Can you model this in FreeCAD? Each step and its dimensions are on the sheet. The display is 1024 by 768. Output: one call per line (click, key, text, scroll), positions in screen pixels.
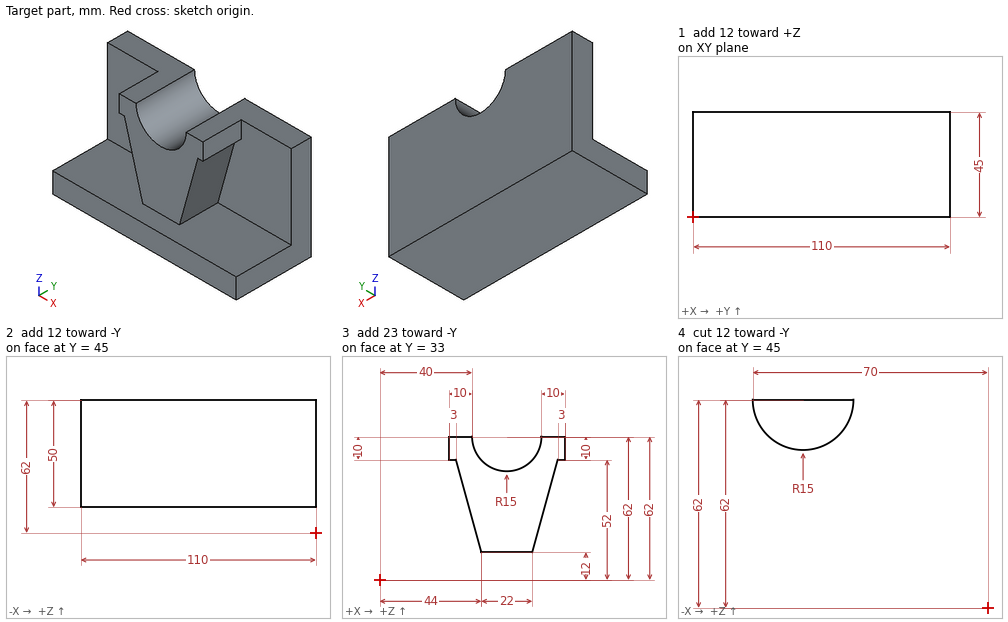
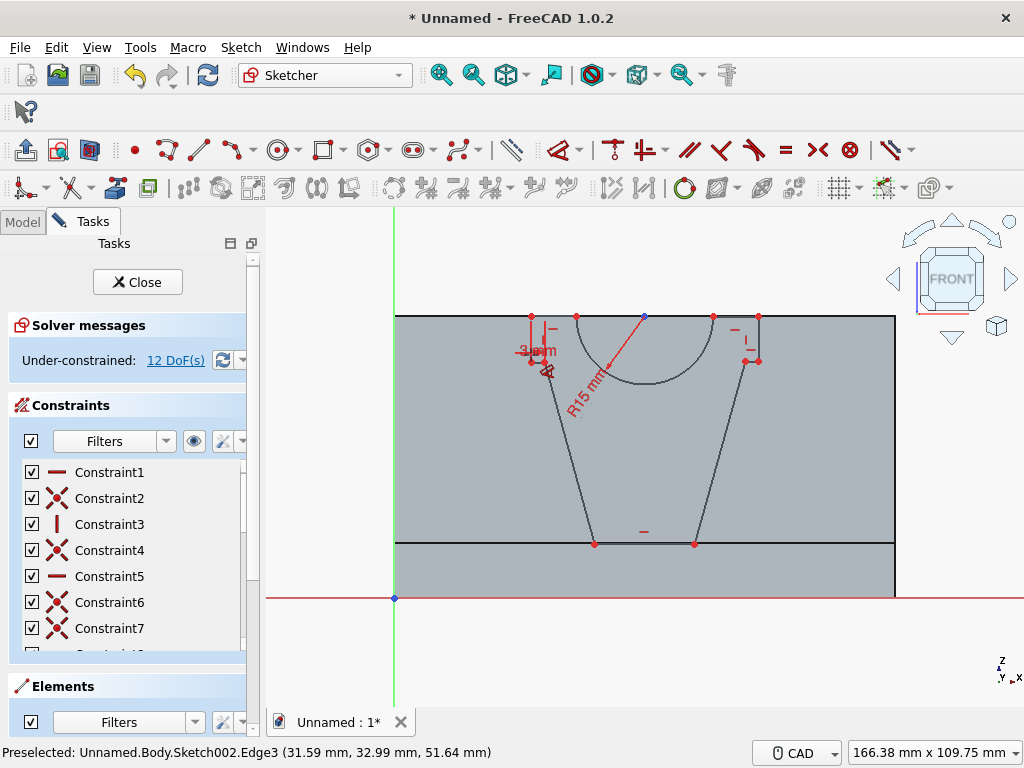
scroll(749, 362, up, 7)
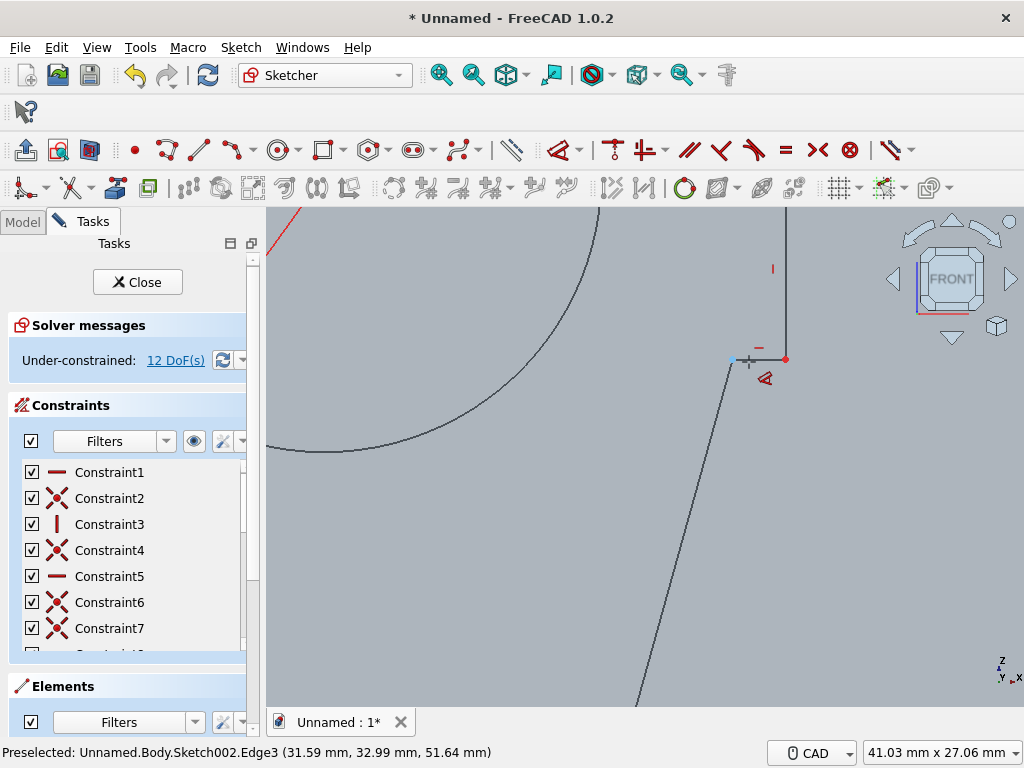
click(748, 360)
click(759, 326)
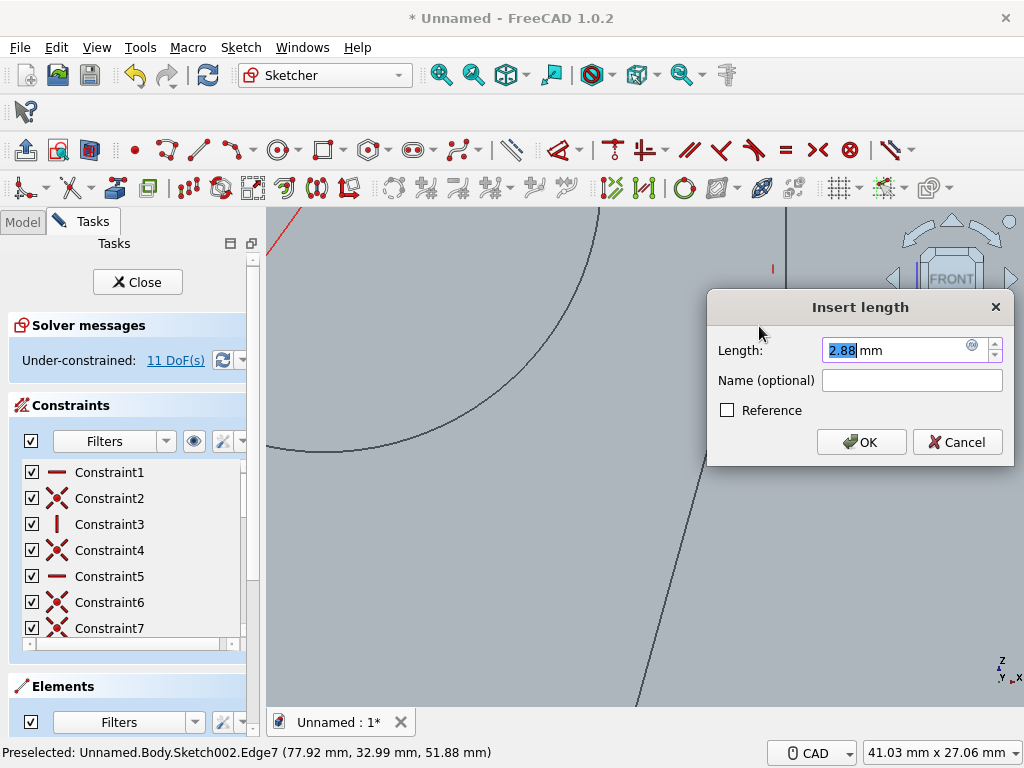
text(3)
key(Return)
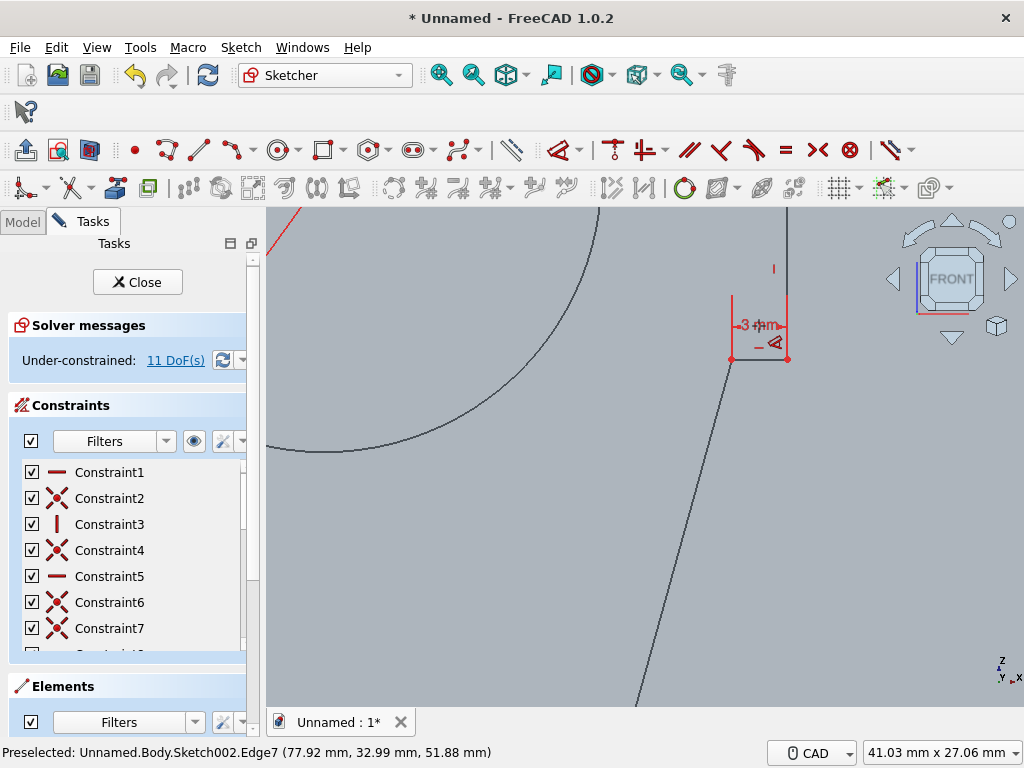
scroll(750, 362, down, 7)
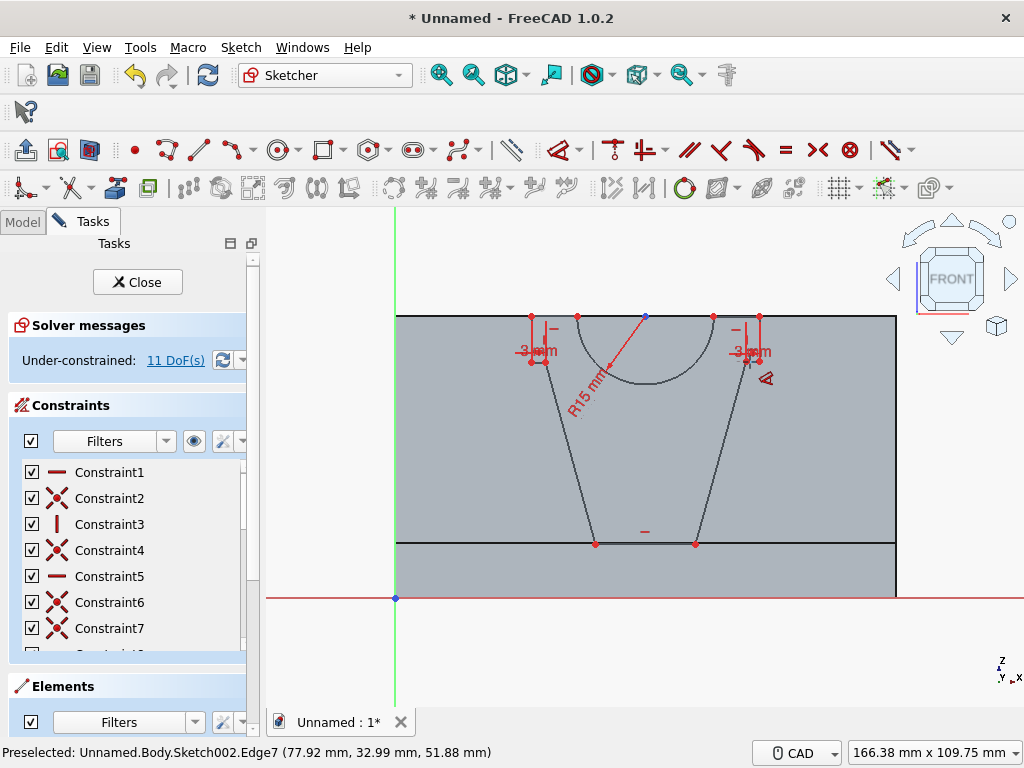
click(564, 316)
click(555, 282)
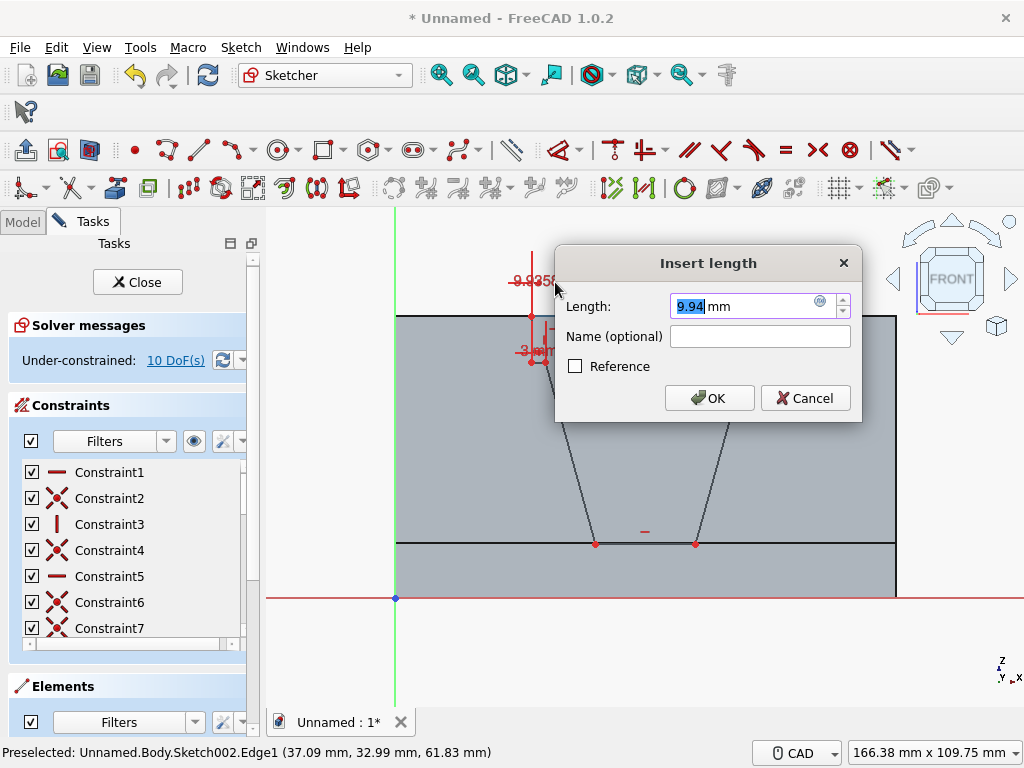
text(10)
key(Return)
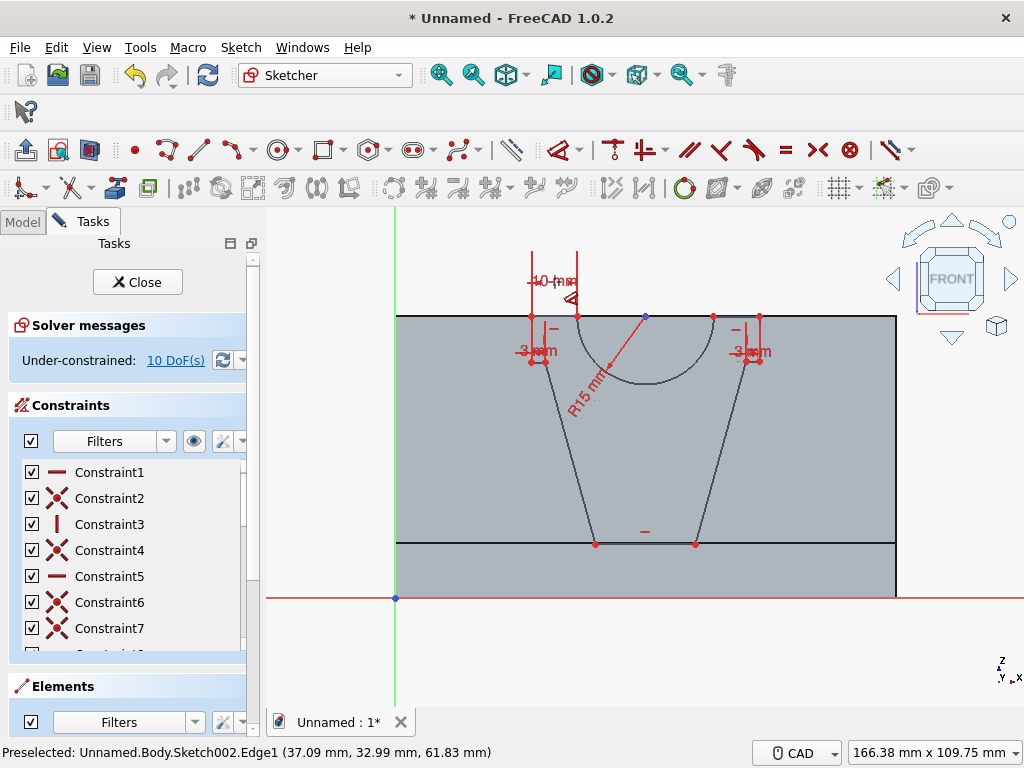
click(532, 330)
click(498, 329)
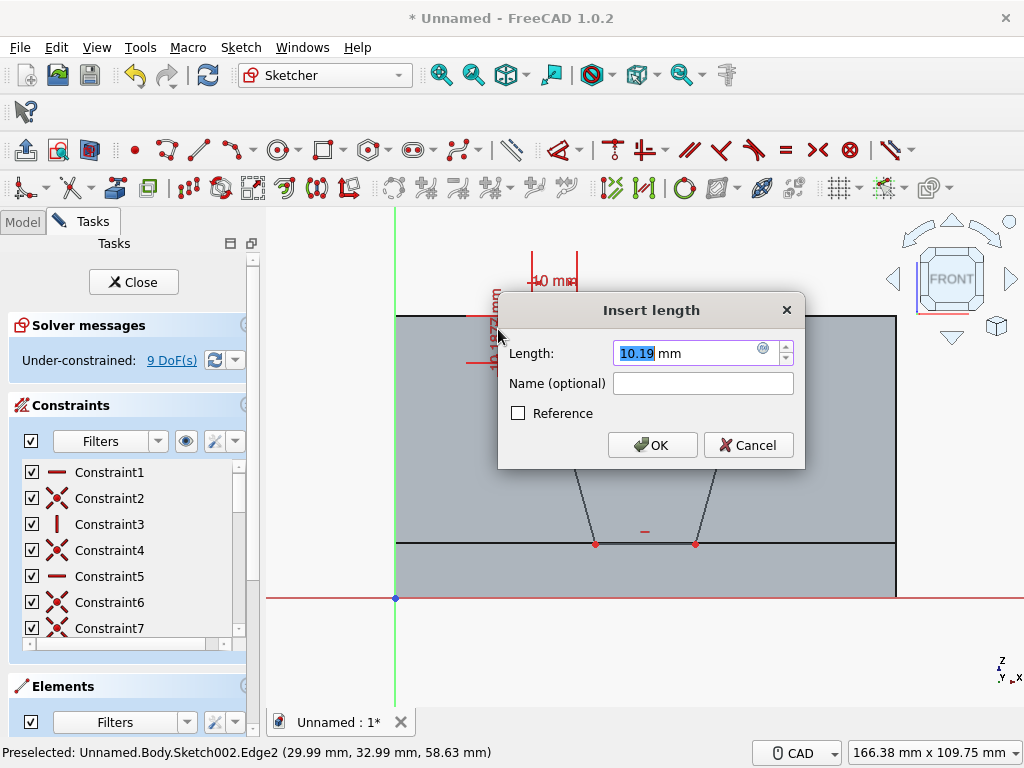
text(10)
key(Return)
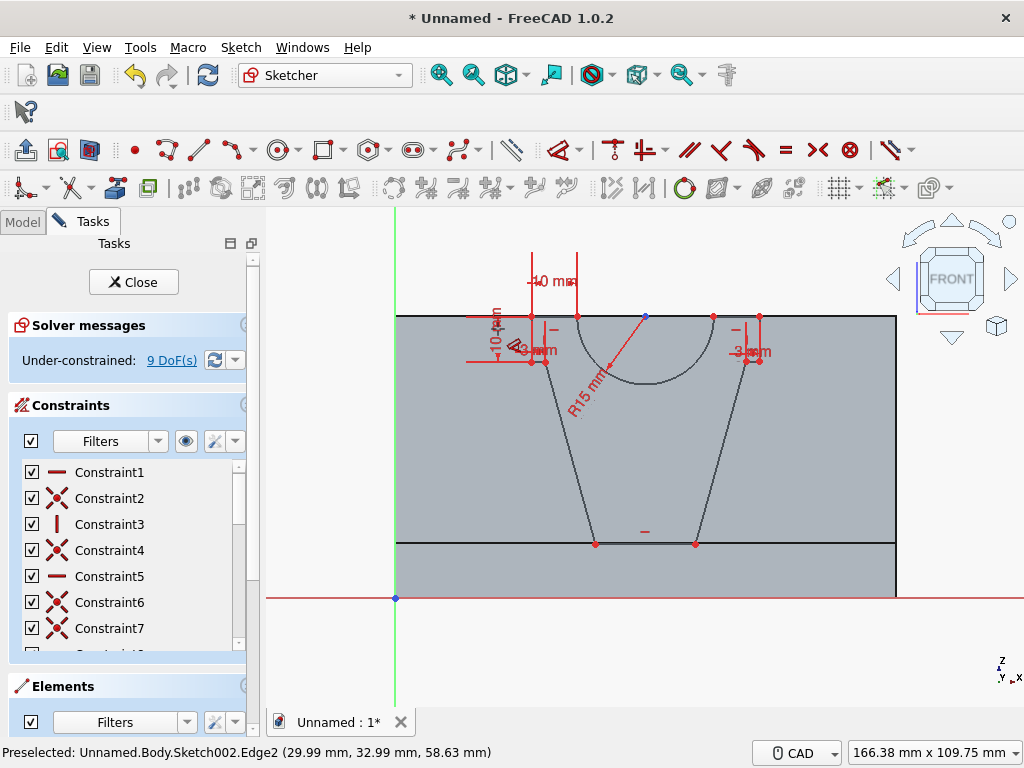
click(625, 544)
click(645, 578)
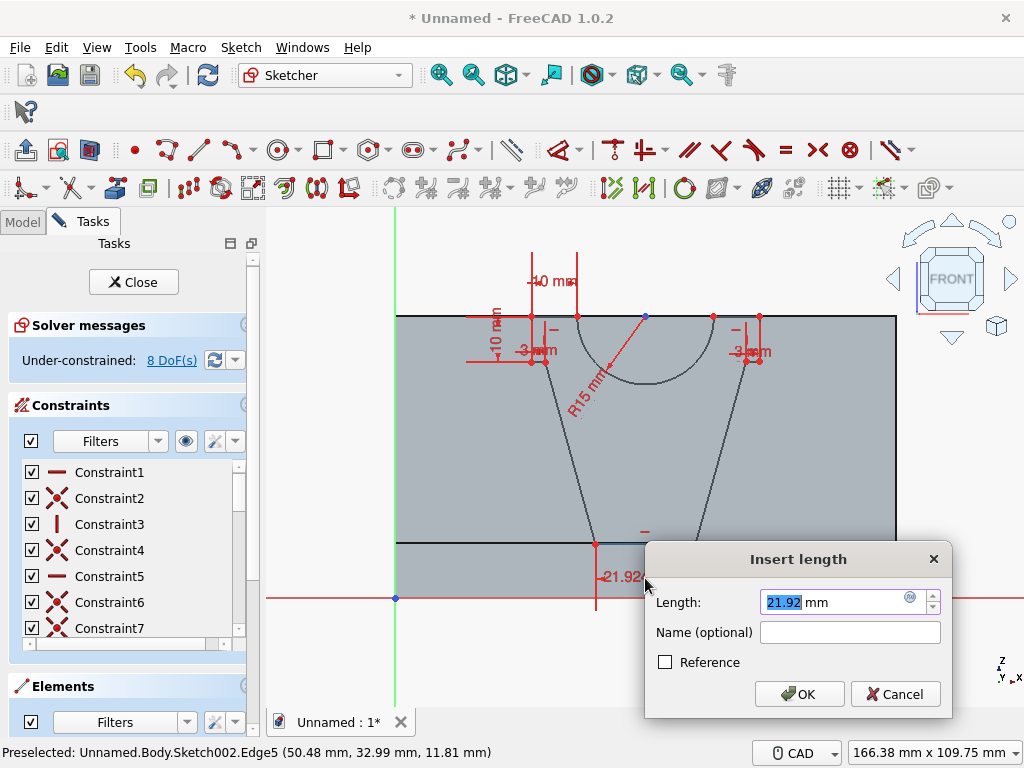
text(22)
key(Return)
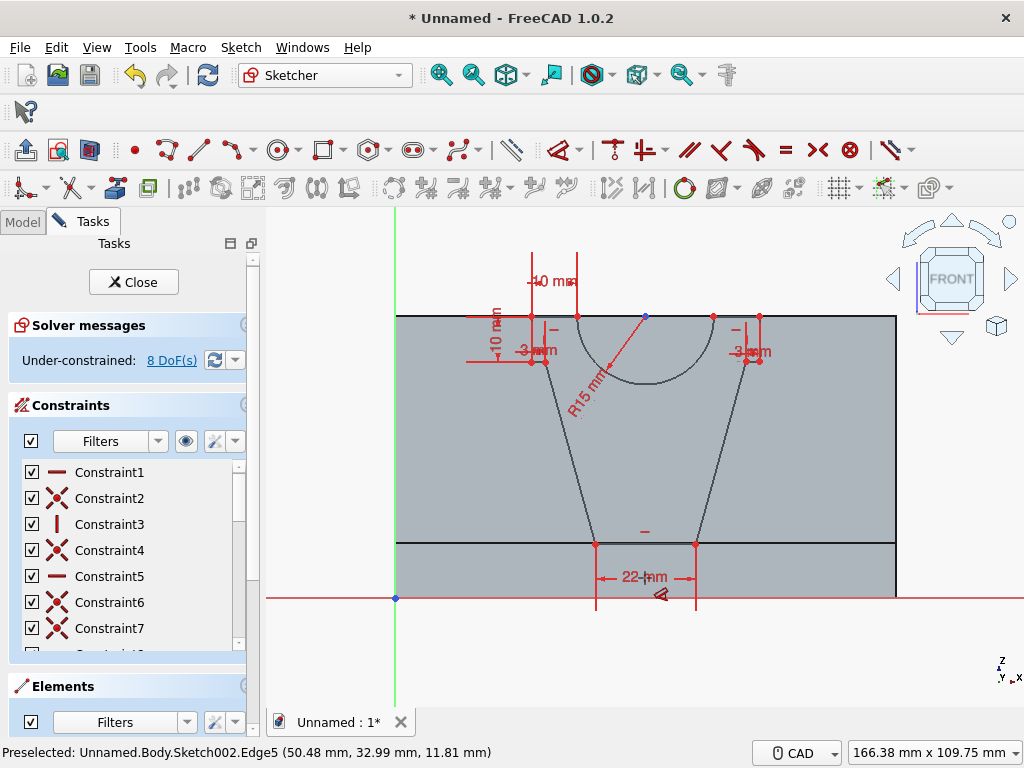
click(760, 348)
click(794, 329)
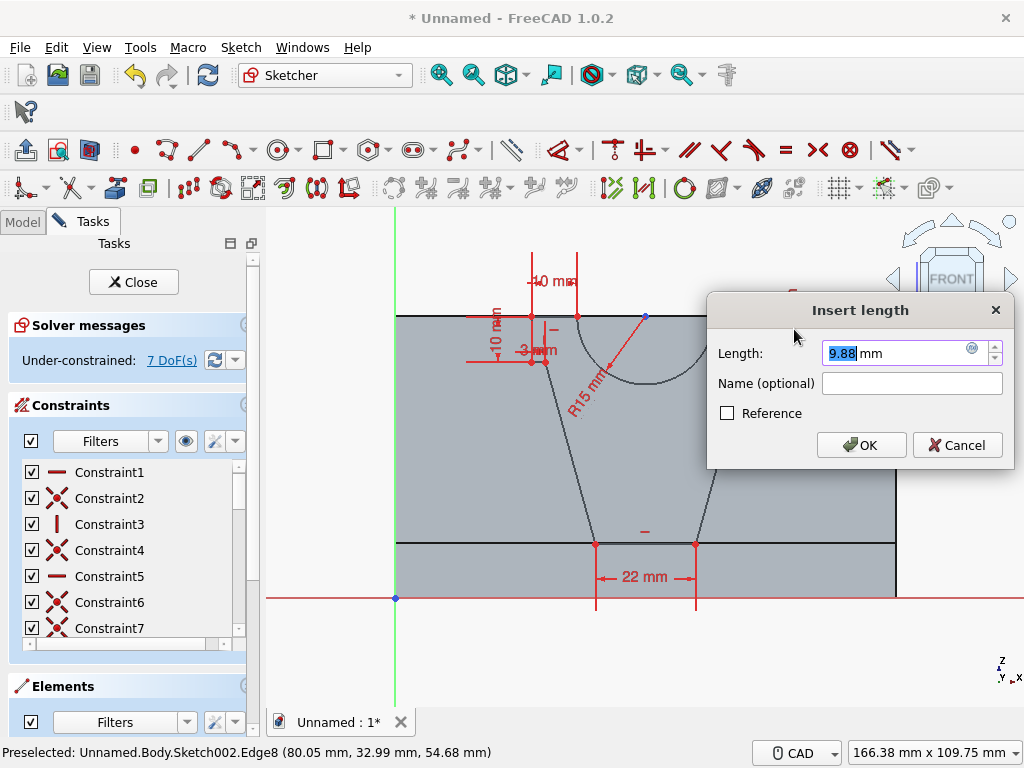
text(10)
key(Return)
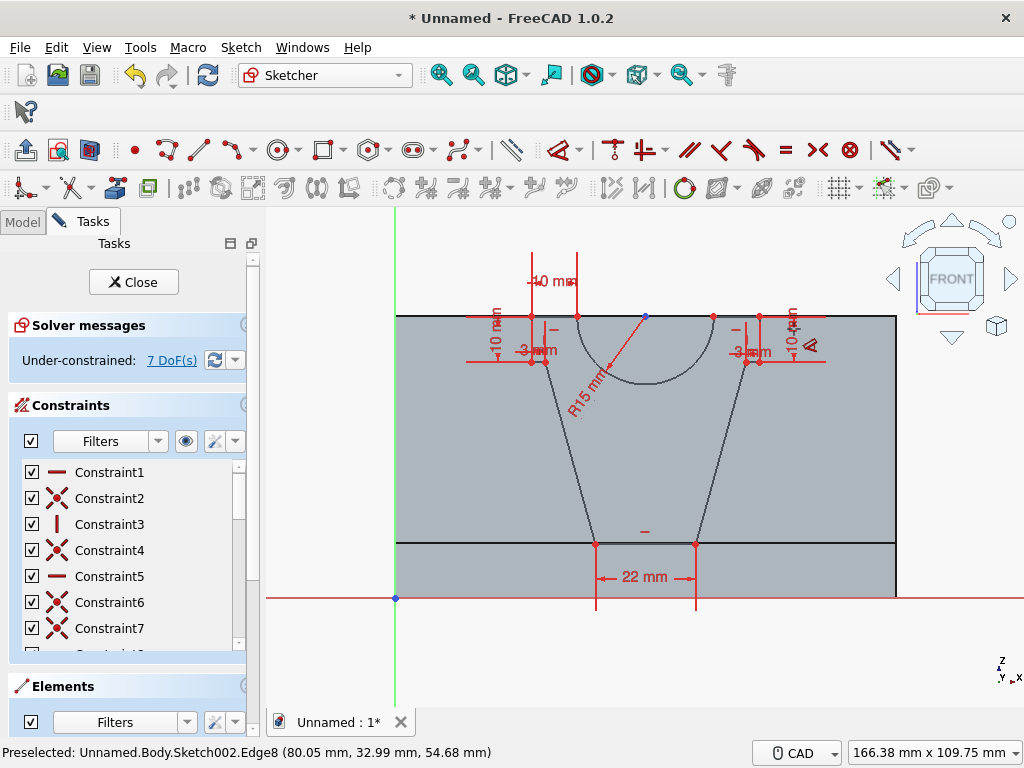
click(746, 317)
click(737, 283)